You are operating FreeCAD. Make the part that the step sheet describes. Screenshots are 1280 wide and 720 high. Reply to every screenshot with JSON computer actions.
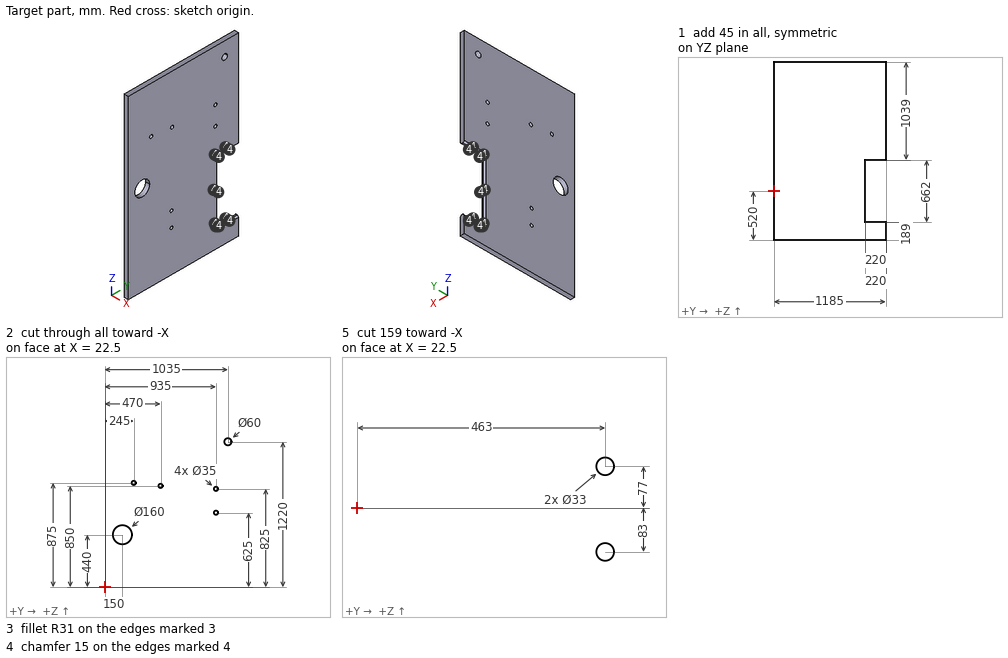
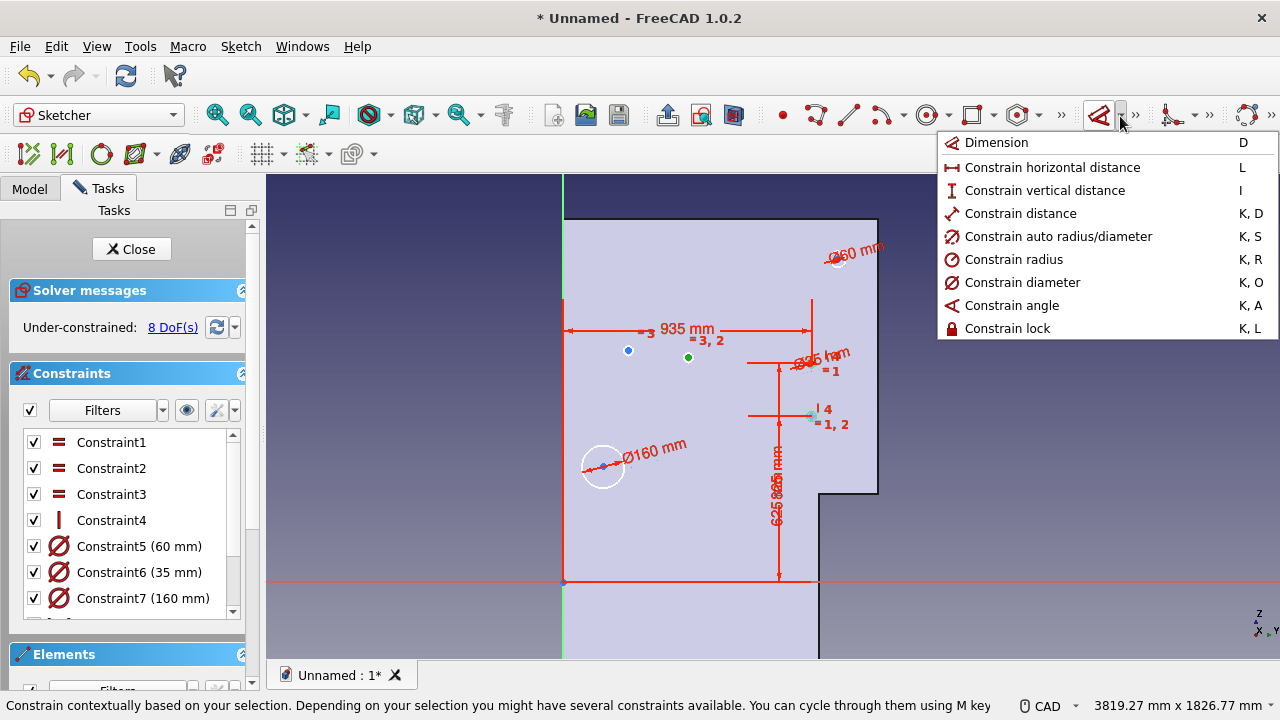
{"action": "left_click", "coordinate": [1108, 168]}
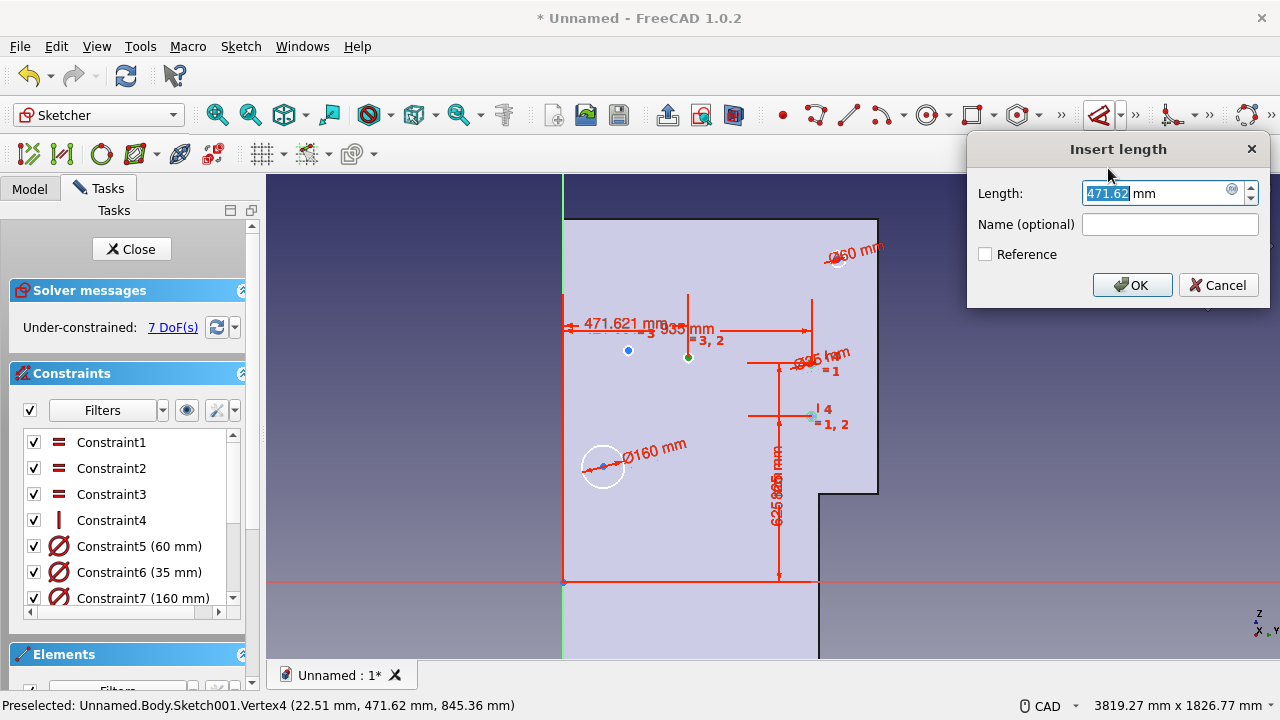
{"action": "type", "text": "470"}
{"action": "key", "text": "Return"}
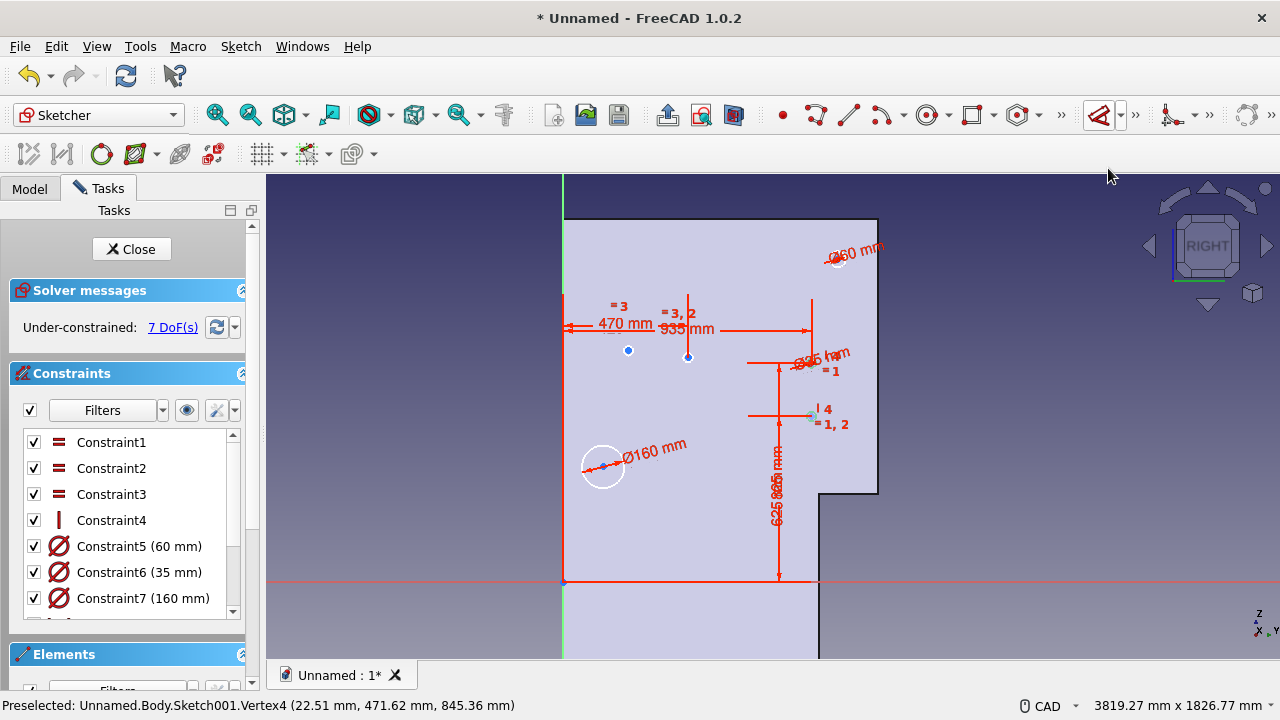
{"action": "left_click", "coordinate": [688, 358]}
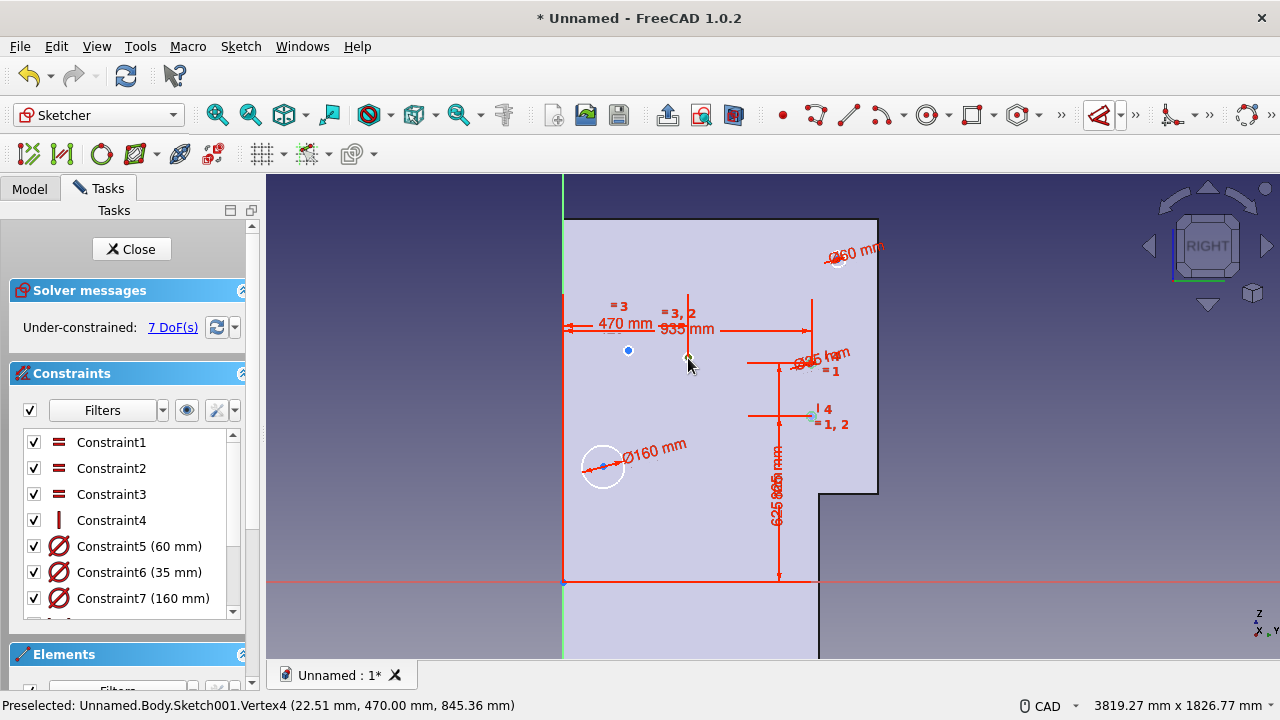
{"action": "left_click", "coordinate": [1120, 116]}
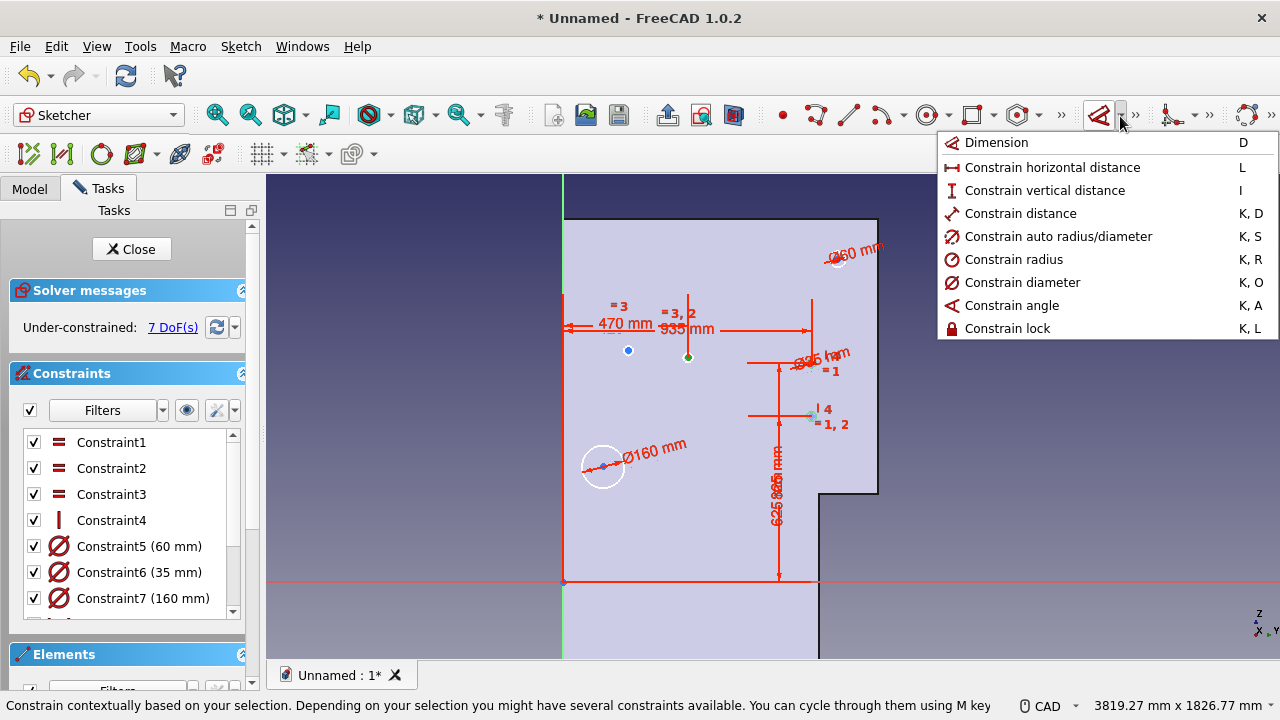
{"action": "left_click", "coordinate": [1108, 190]}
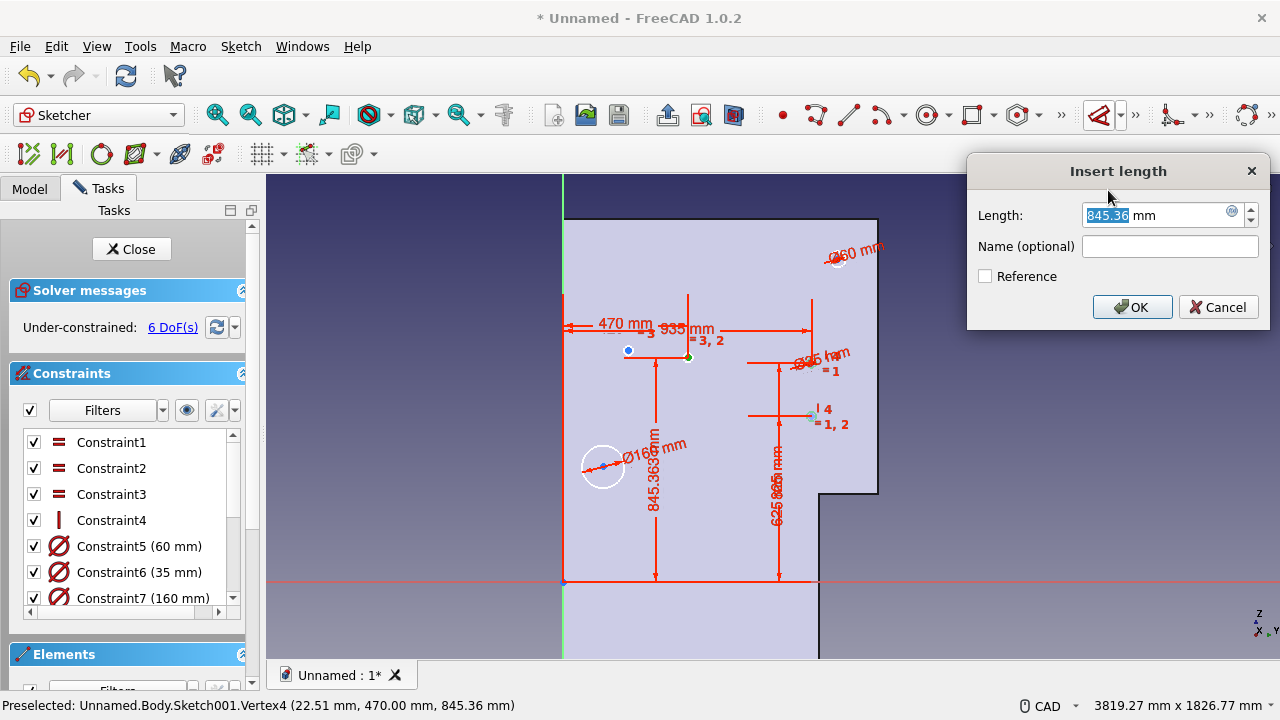
{"action": "type", "text": "850"}
{"action": "key", "text": "Return"}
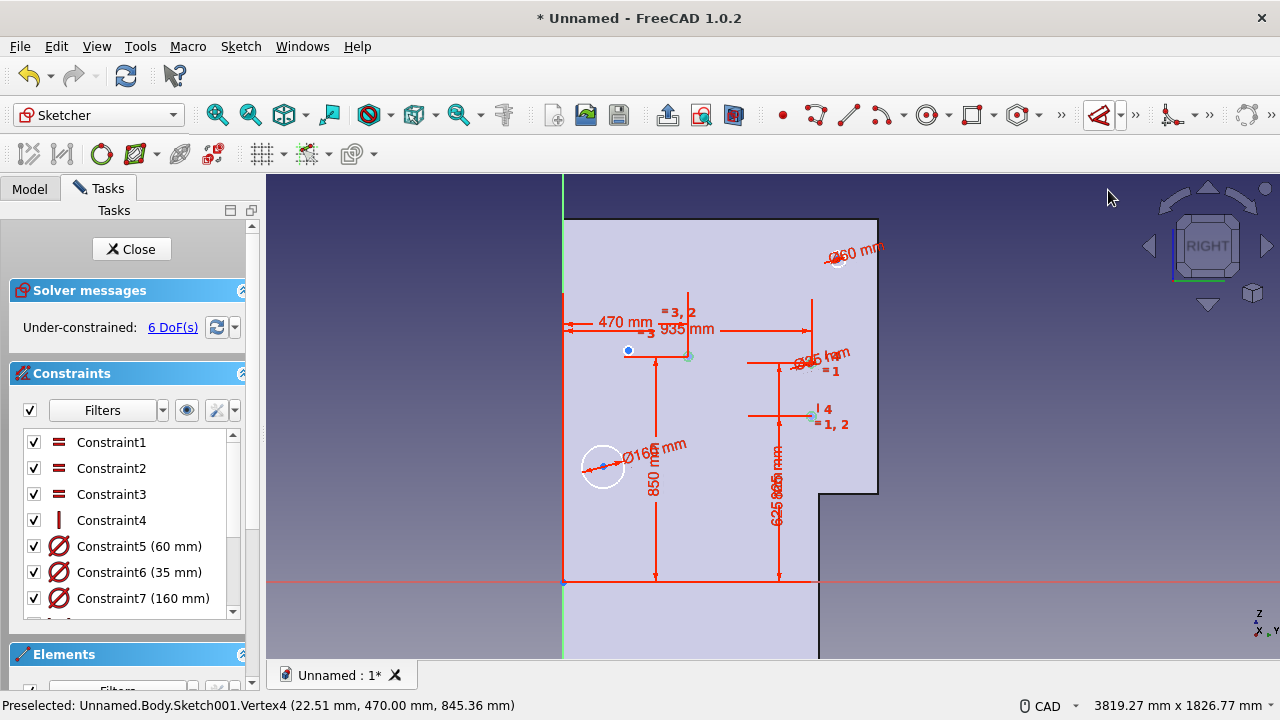
{"action": "left_click", "coordinate": [629, 351]}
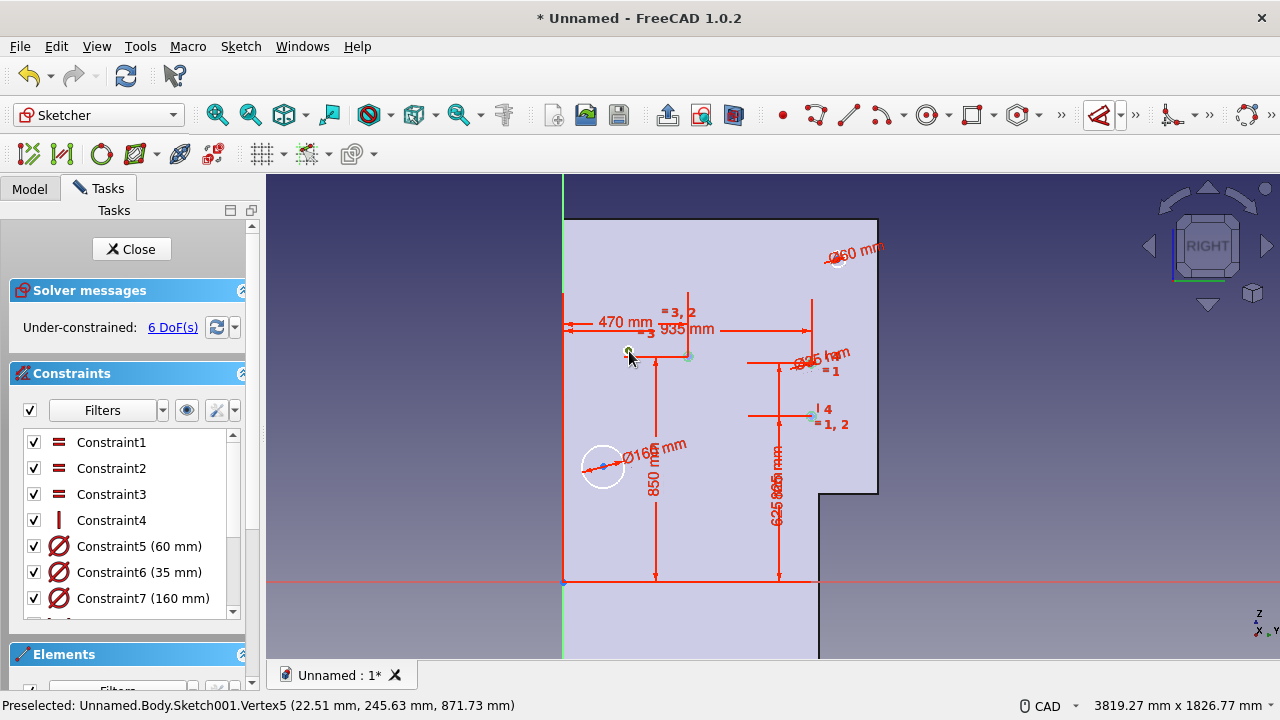
{"action": "left_click", "coordinate": [1120, 116]}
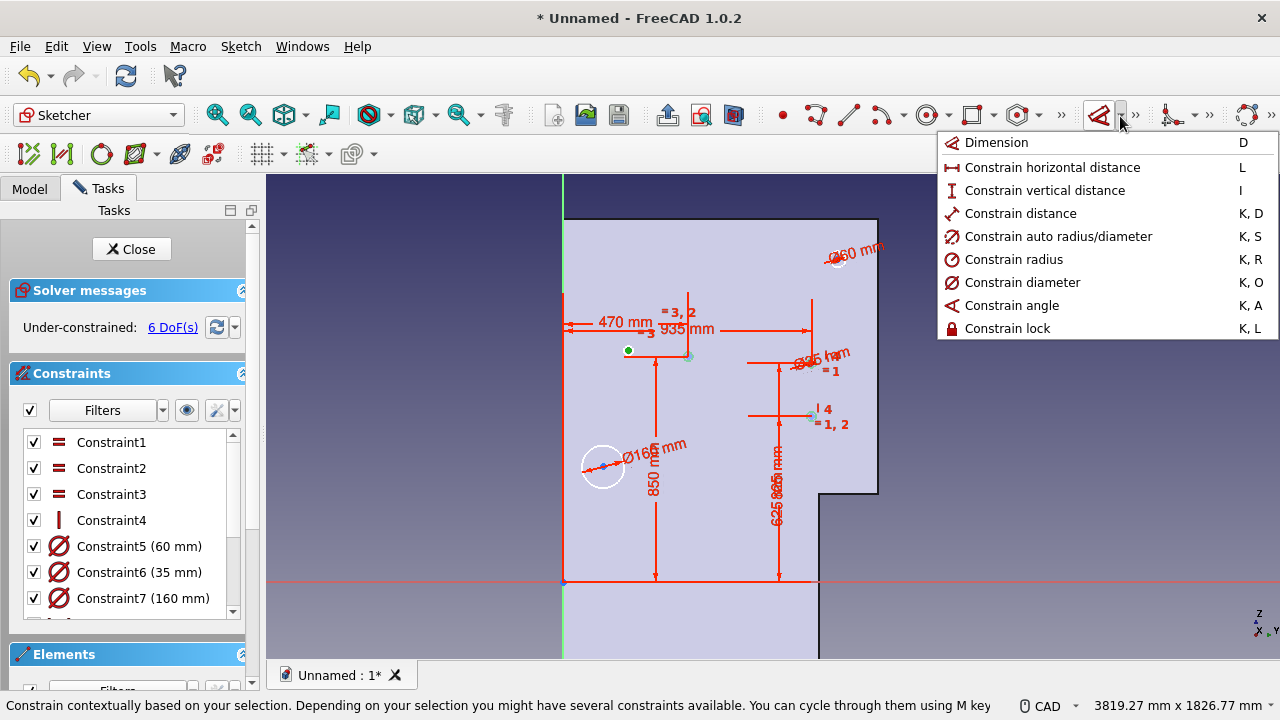
{"action": "left_click", "coordinate": [1108, 168]}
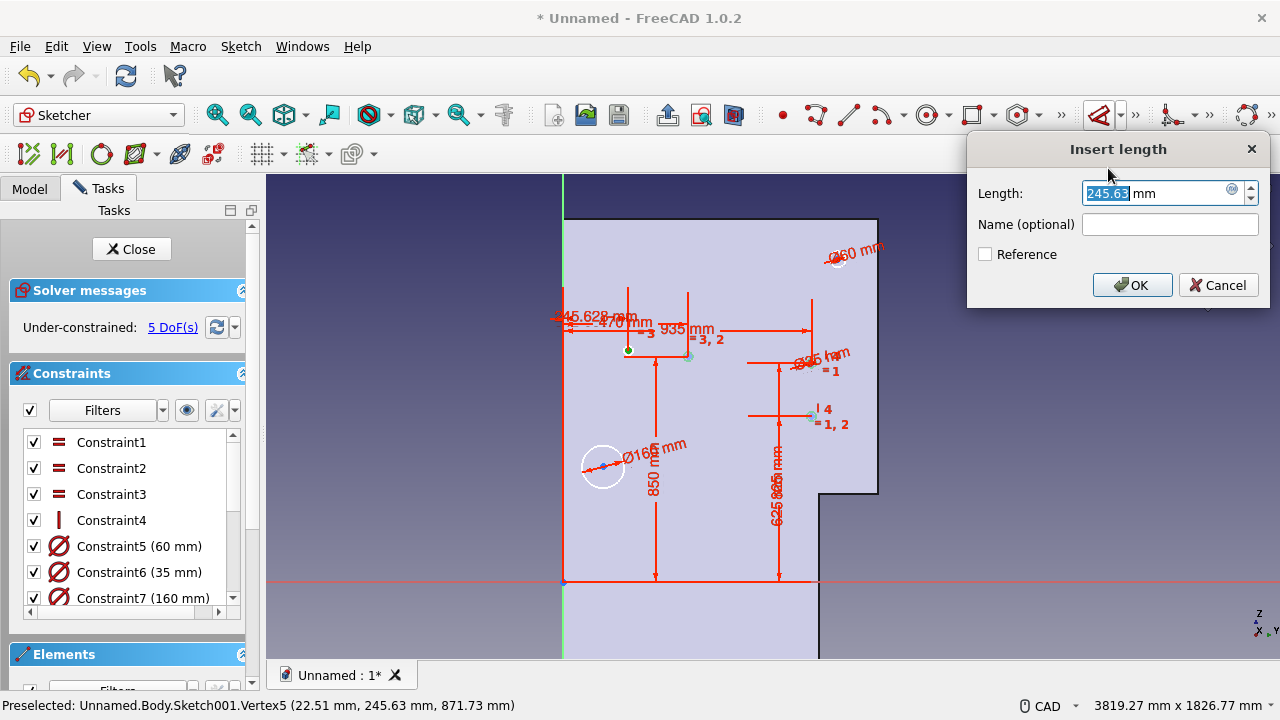
{"action": "type", "text": "245"}
{"action": "key", "text": "Return"}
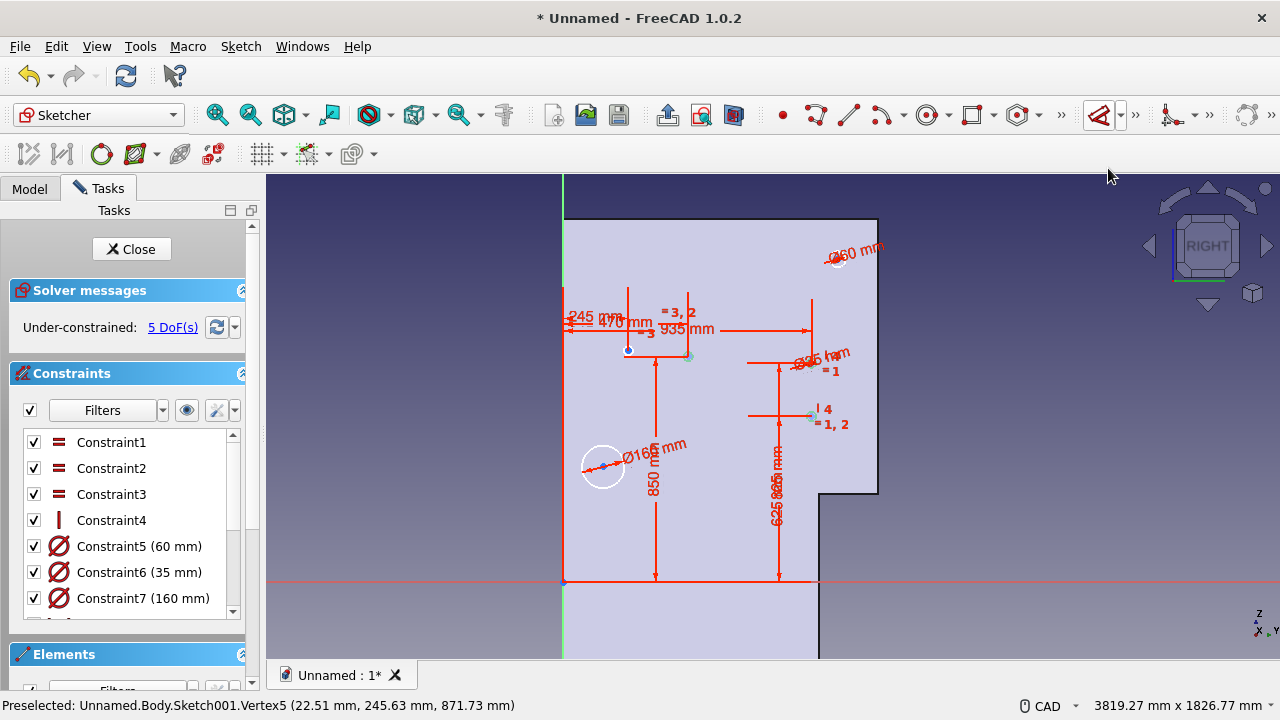
{"action": "left_click", "coordinate": [628, 351]}